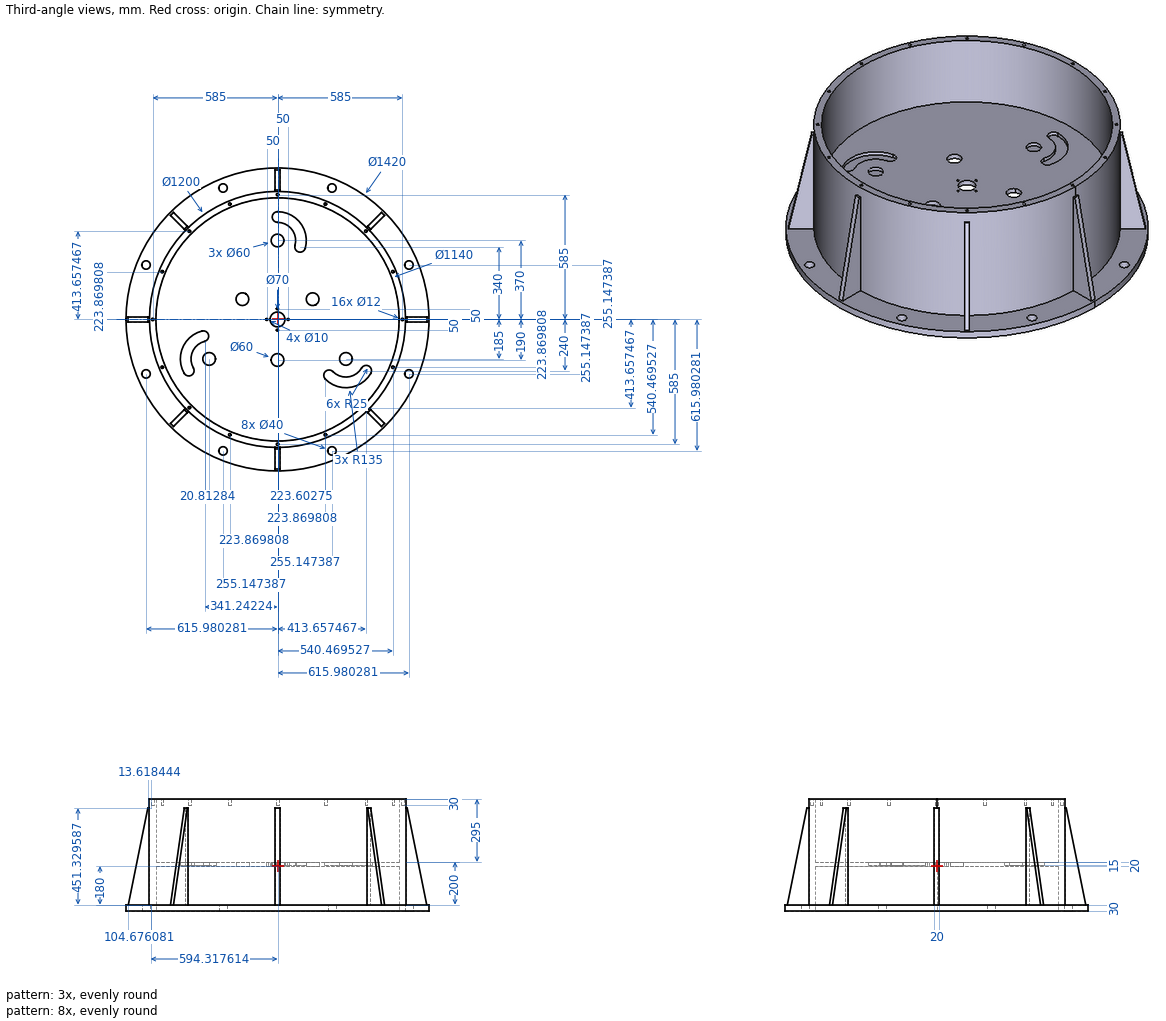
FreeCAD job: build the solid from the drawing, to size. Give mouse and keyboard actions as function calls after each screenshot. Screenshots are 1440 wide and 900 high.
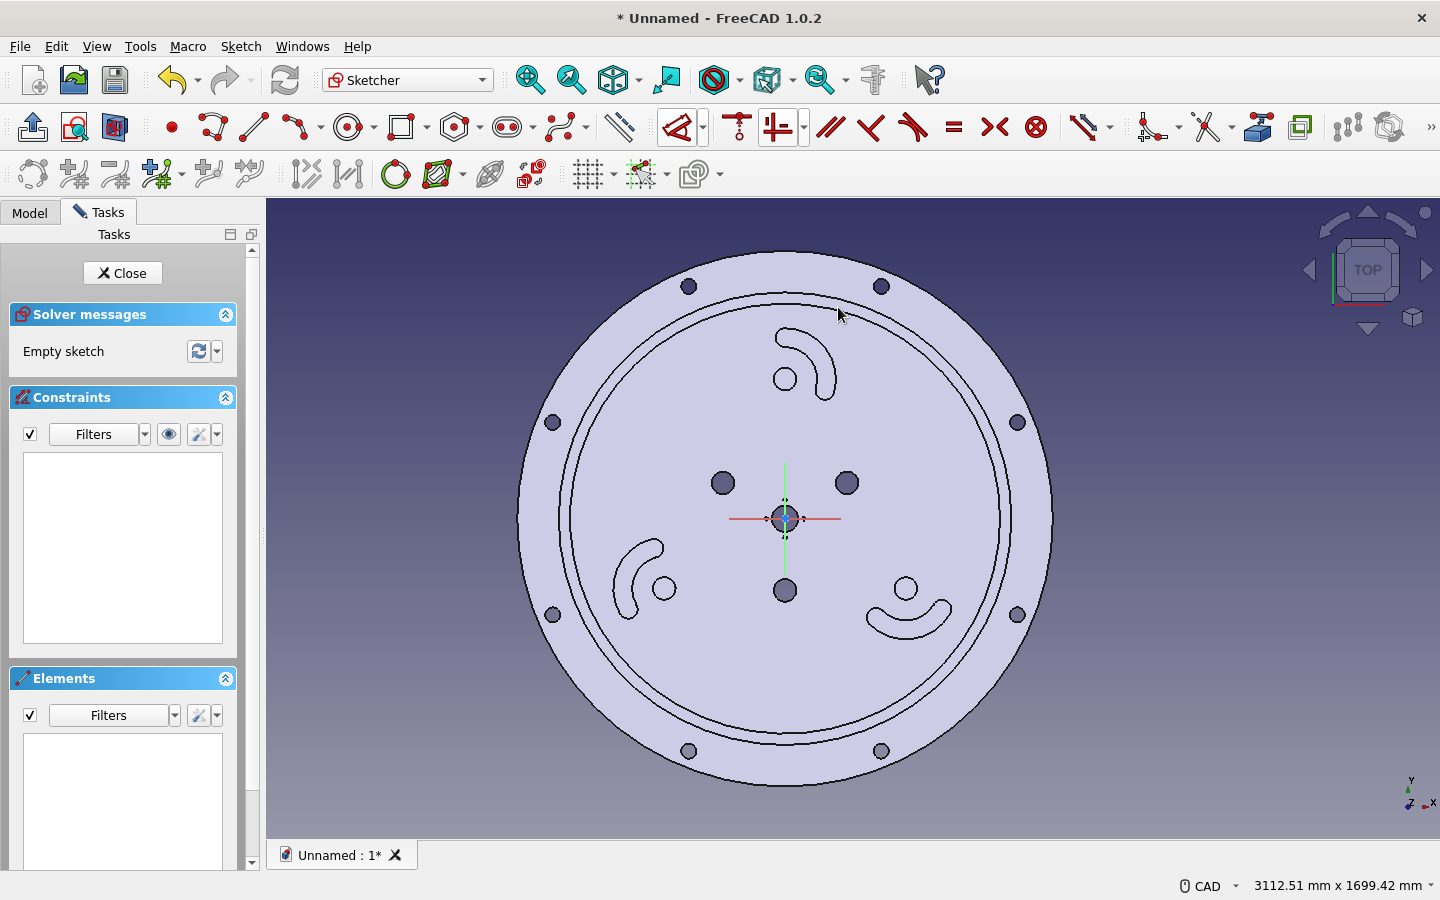
click(348, 128)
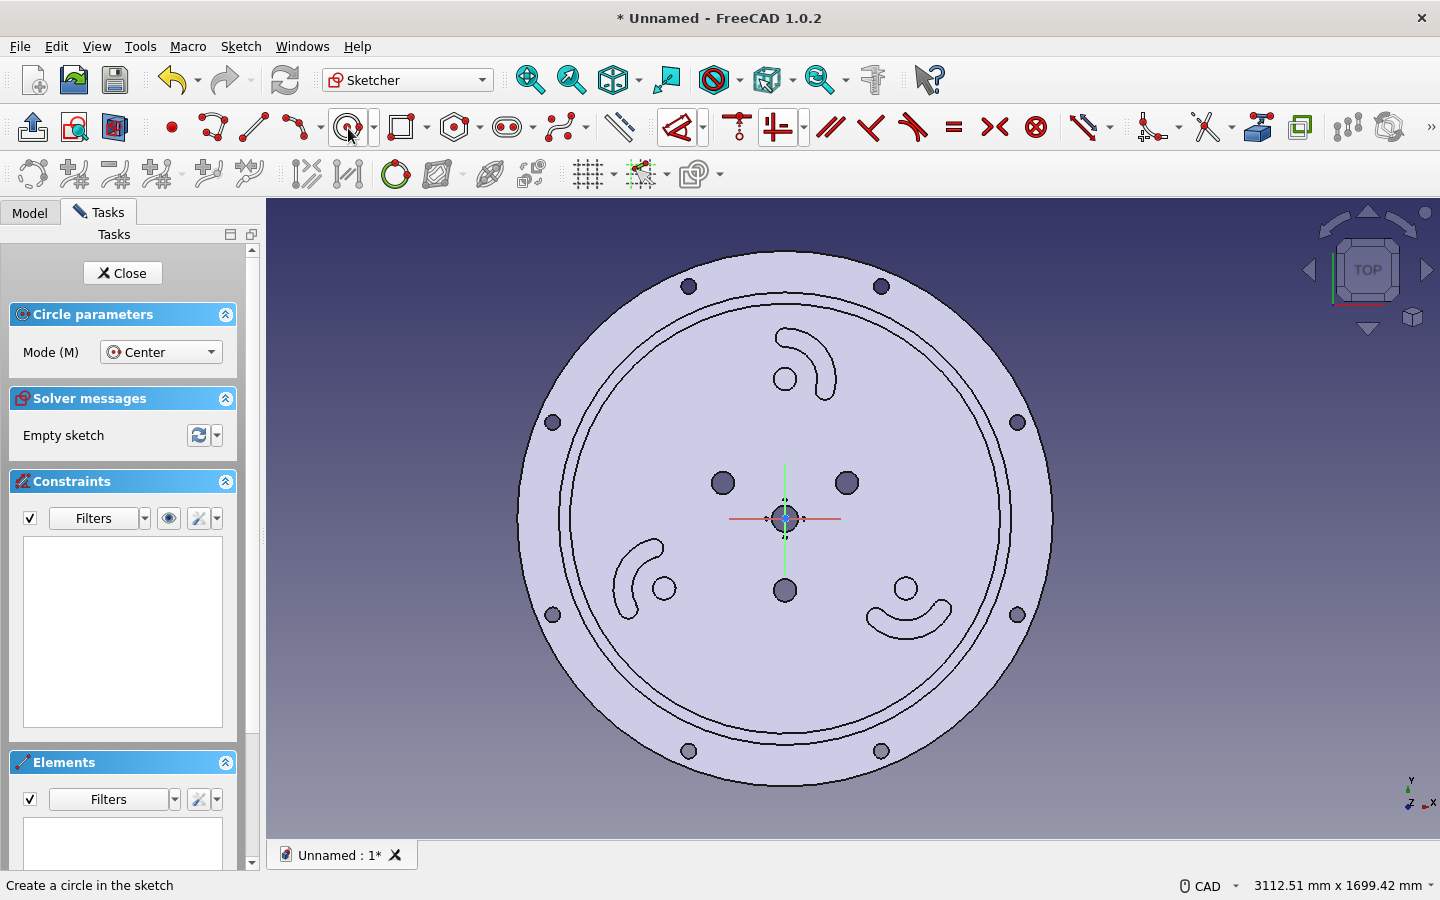
scroll(1006, 519, up, 12)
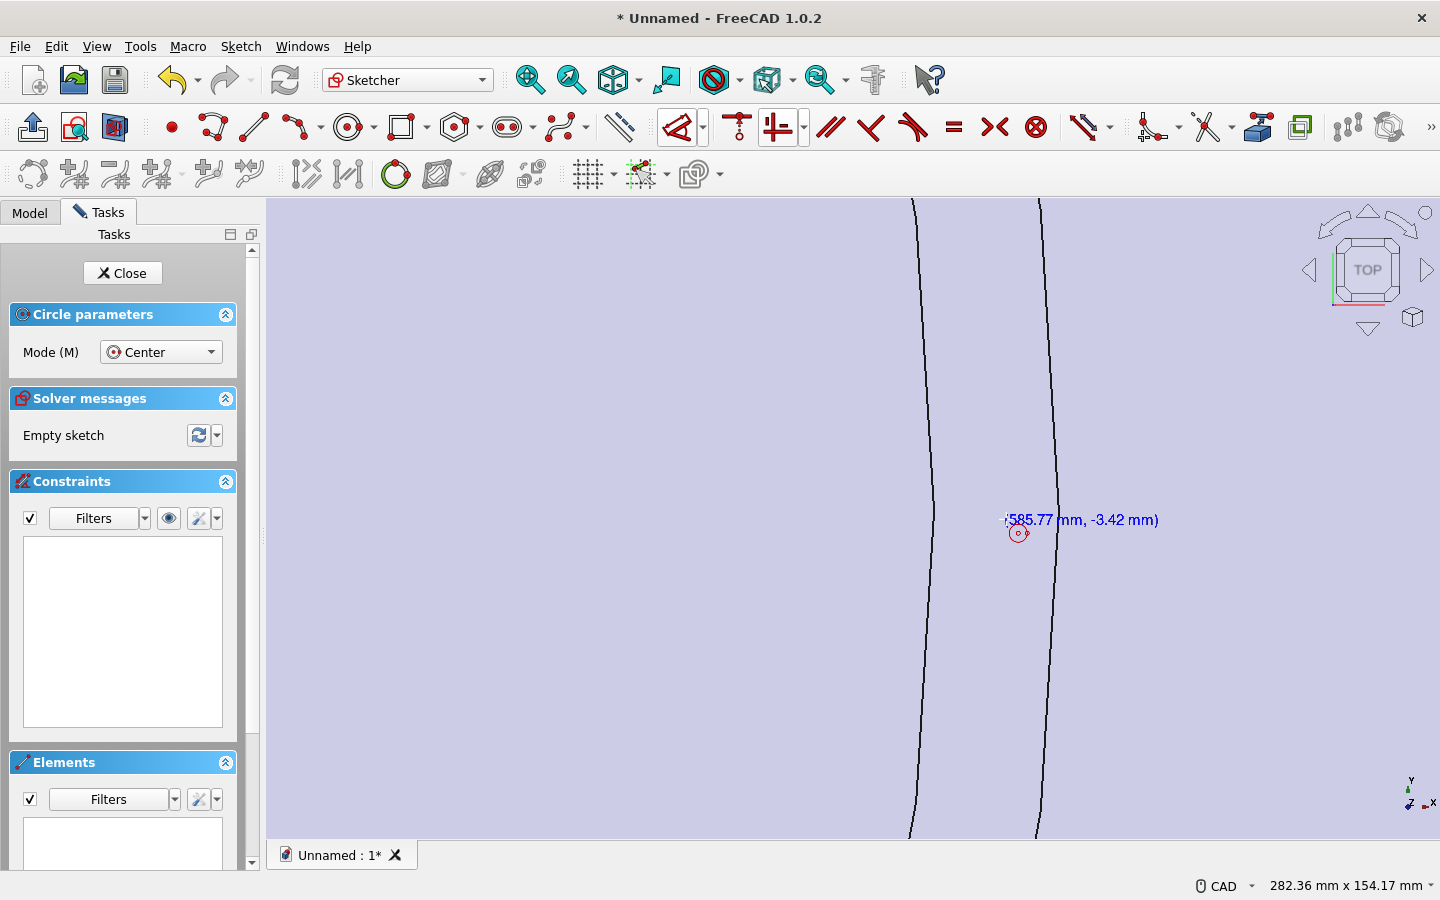
scroll(1006, 519, down, 12)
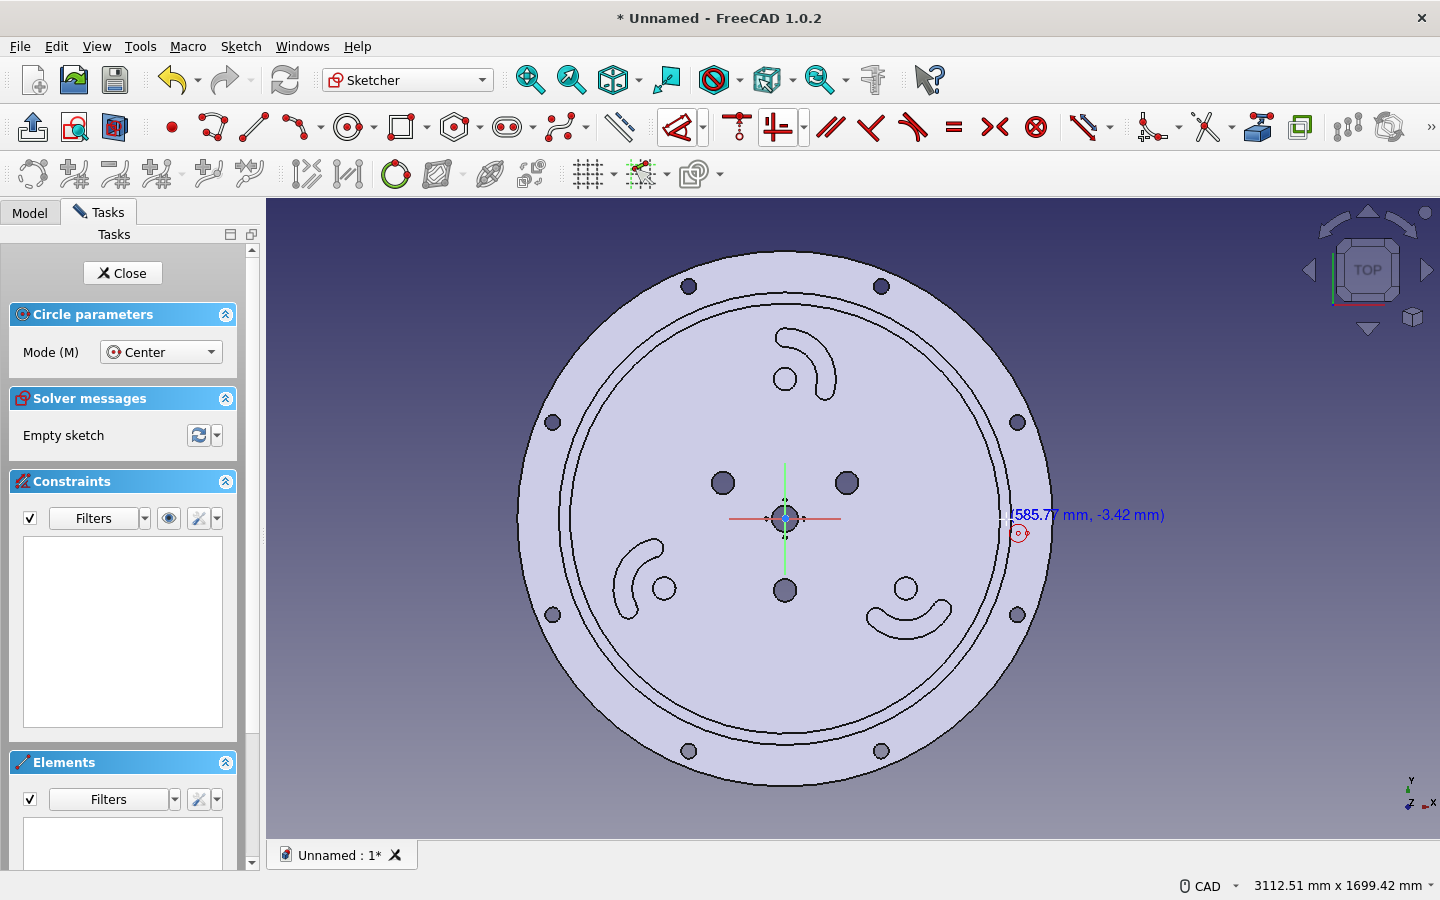
click(1006, 519)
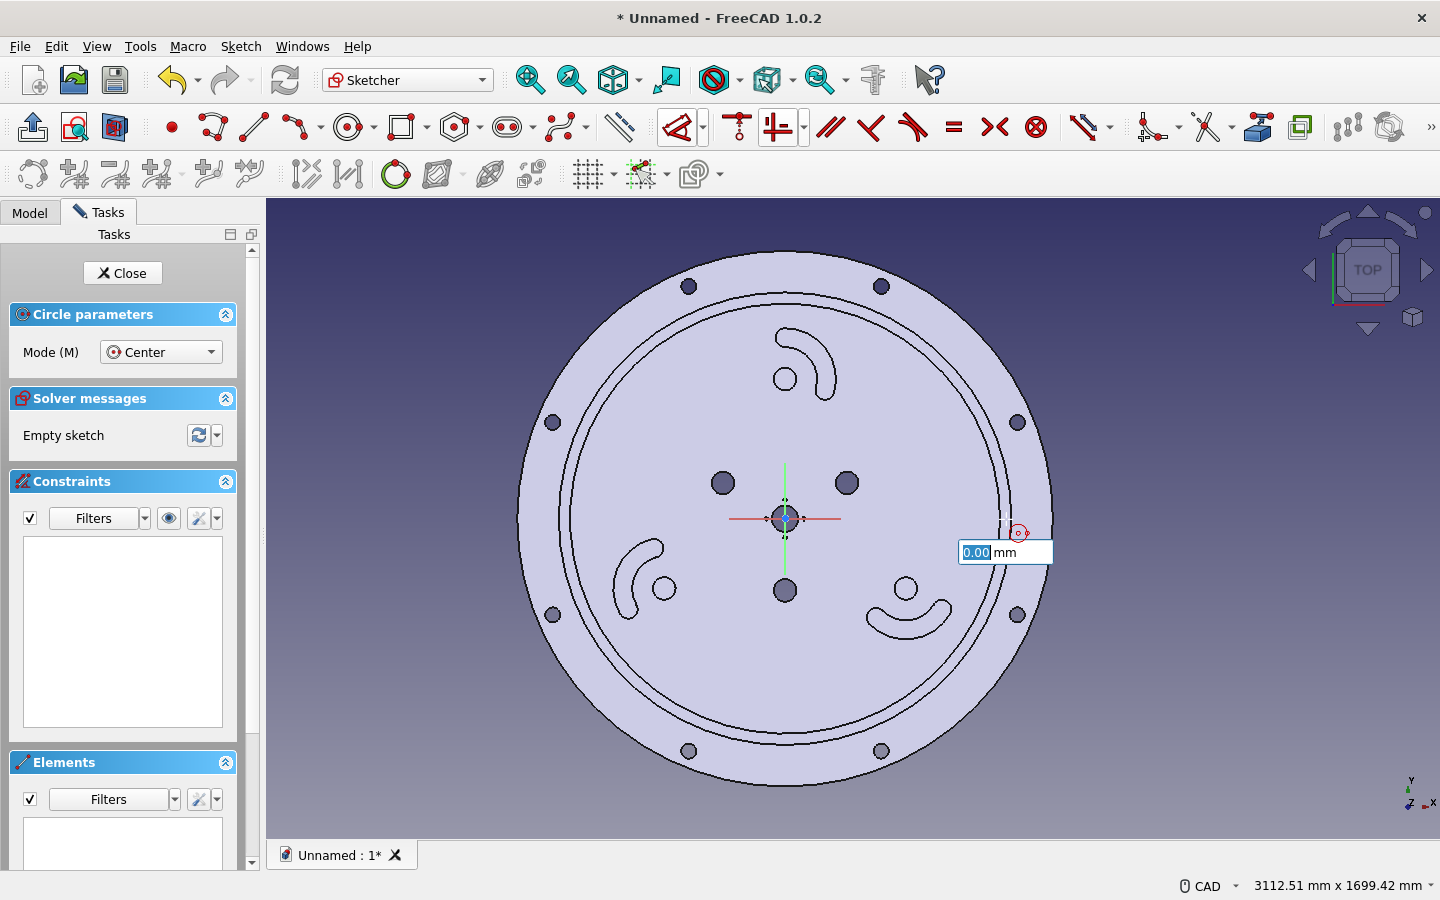
scroll(1005, 521, up, 11)
move(999, 515)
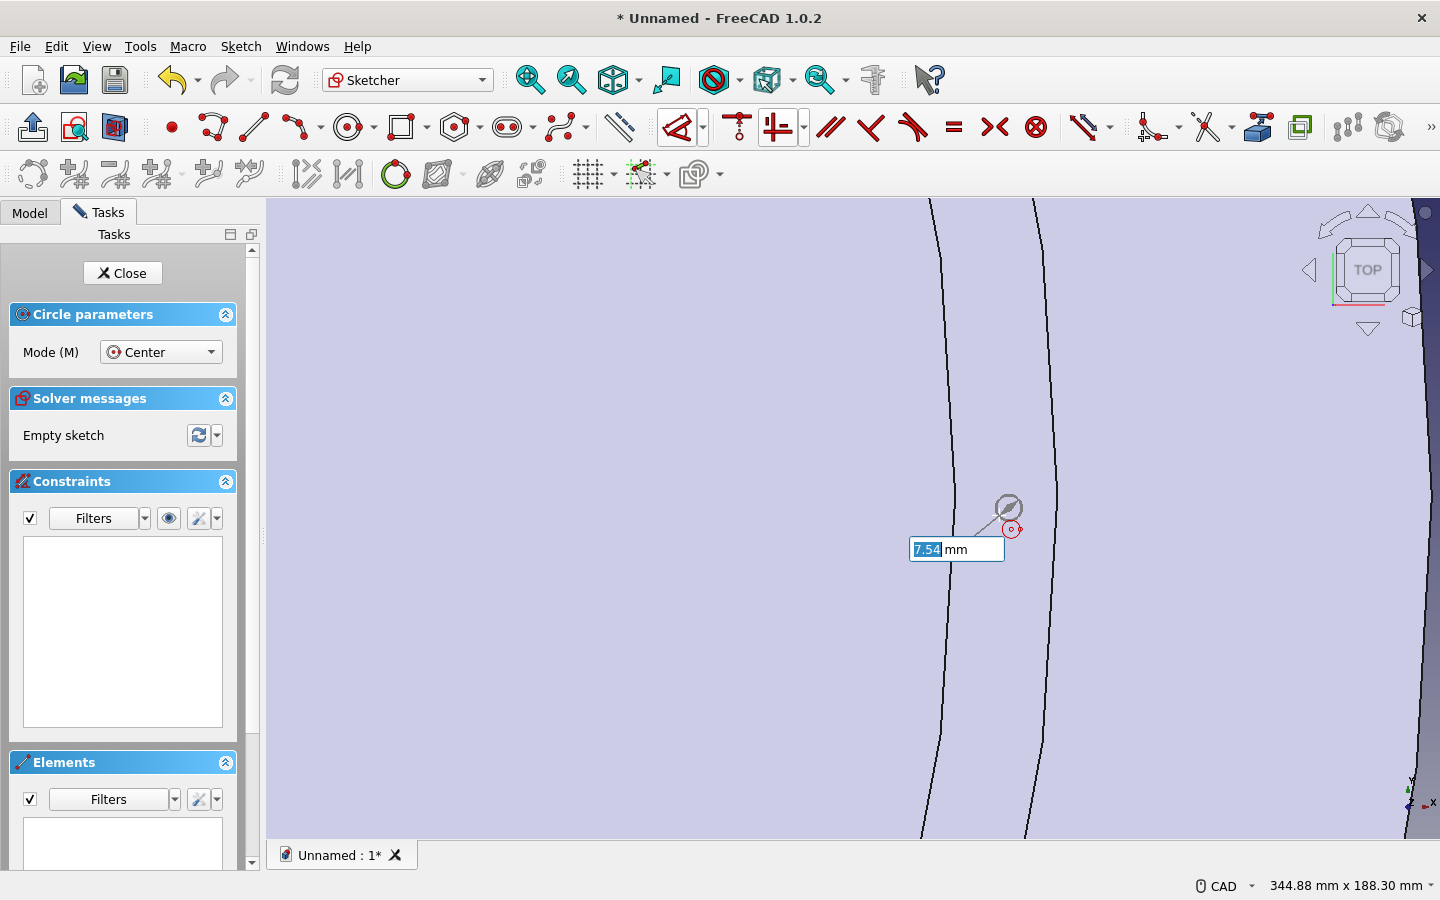
text(12)
key(Return)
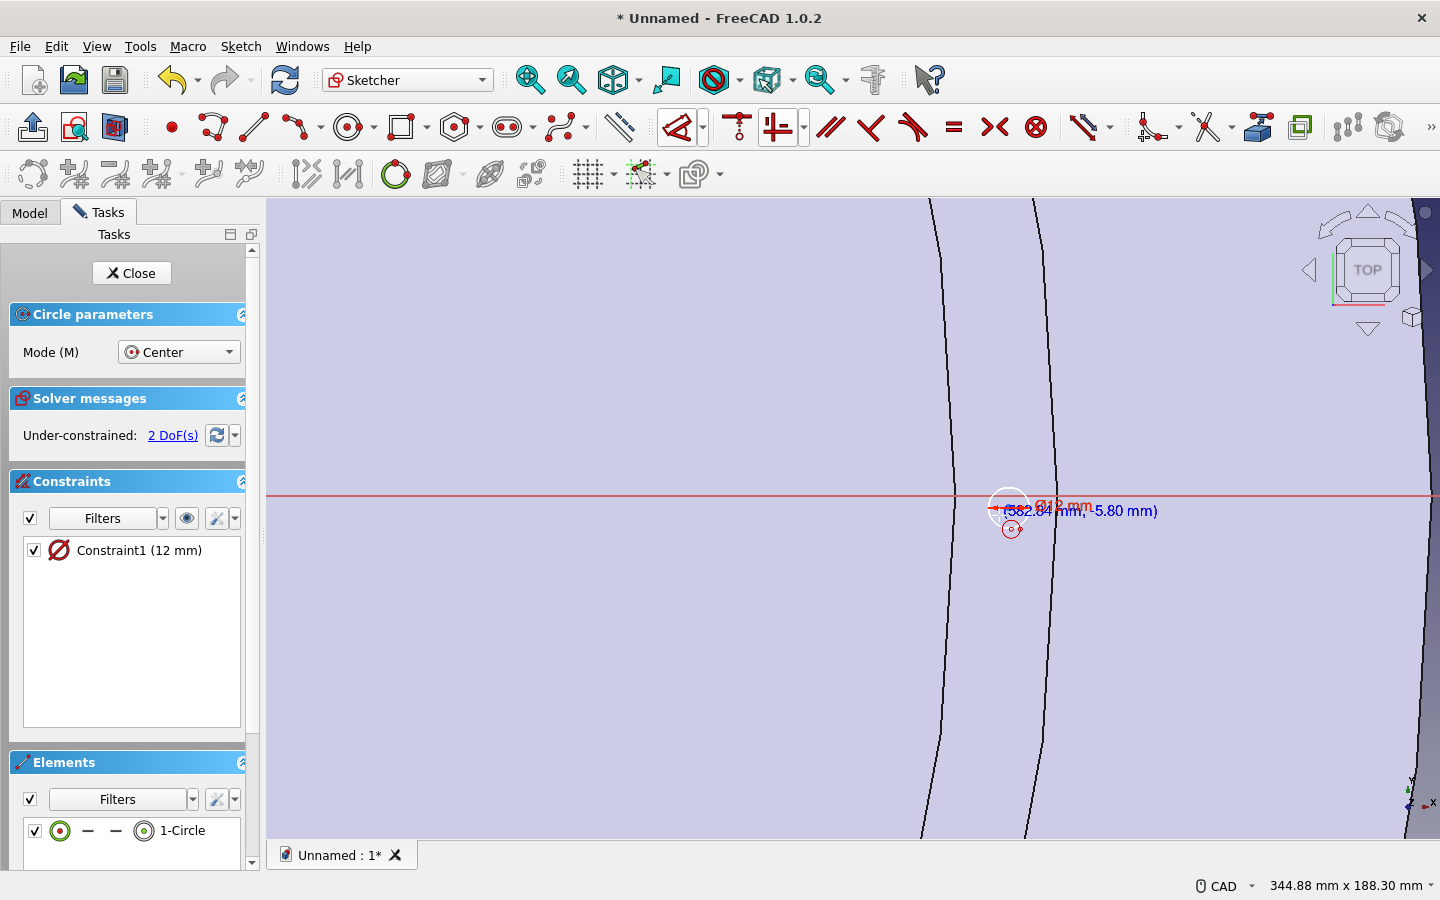
scroll(1005, 521, down, 11)